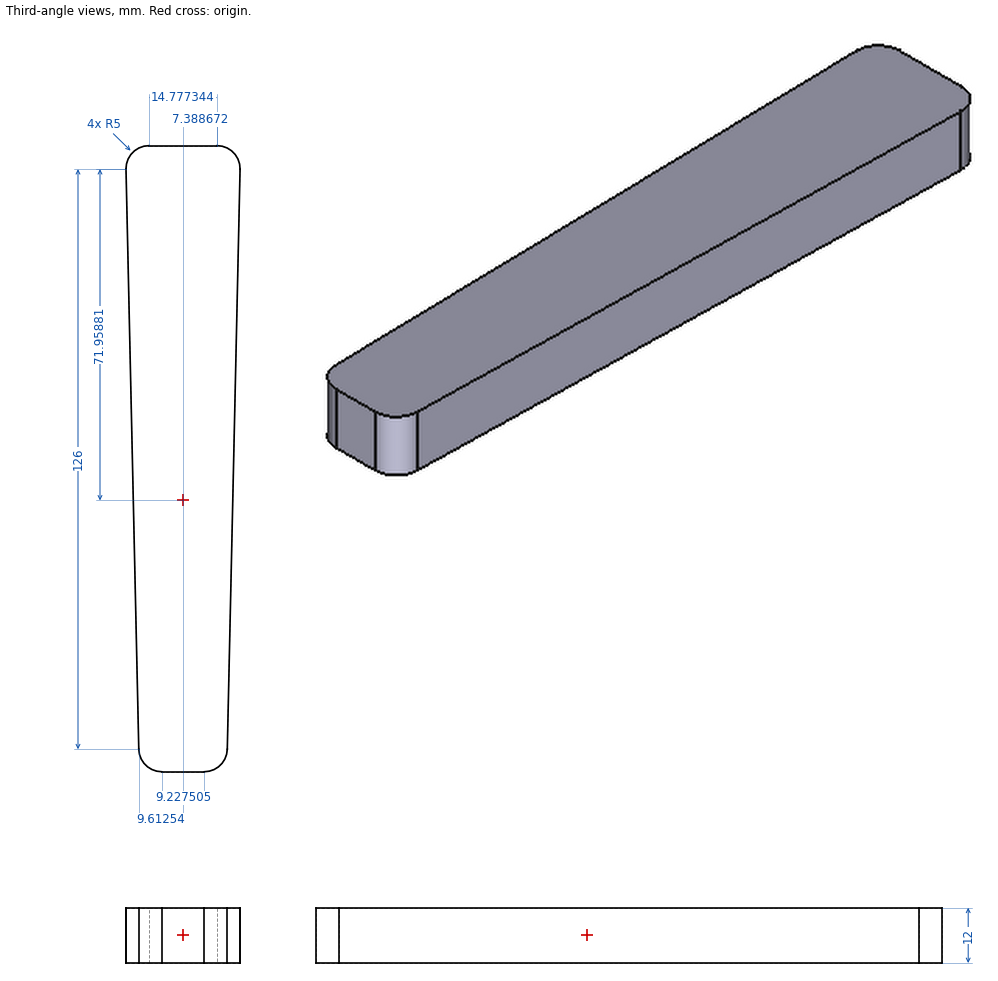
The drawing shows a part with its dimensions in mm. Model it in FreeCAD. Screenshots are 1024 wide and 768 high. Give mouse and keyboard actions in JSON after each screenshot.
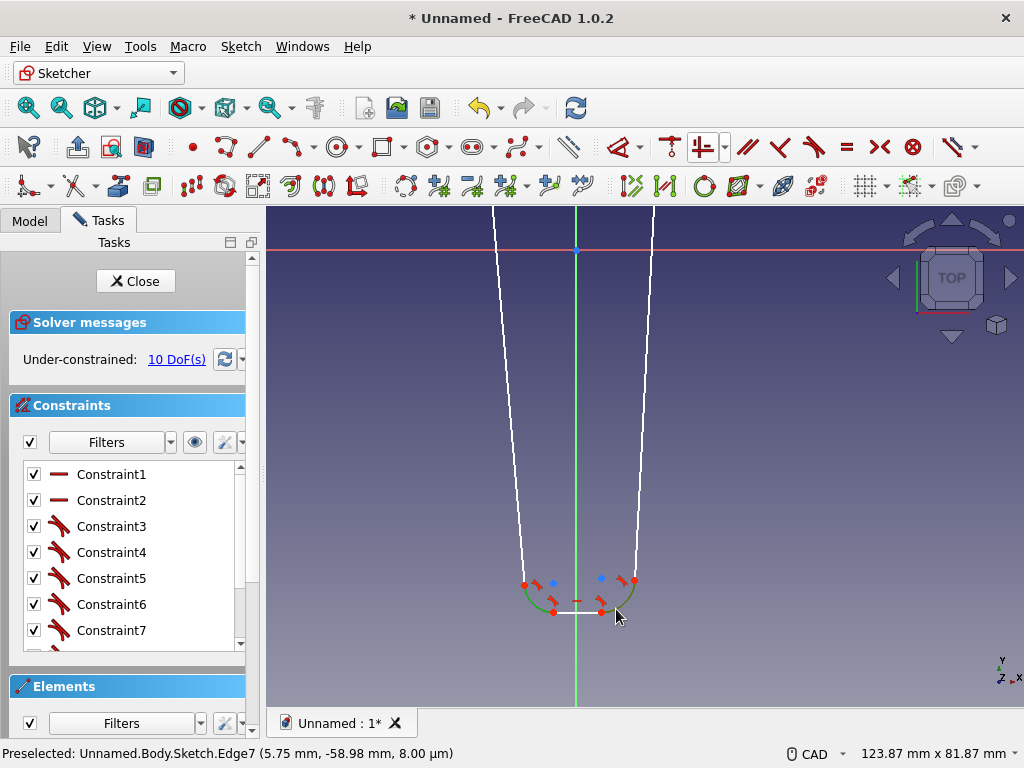
{"action": "scroll", "coordinate": [577, 609], "scroll_direction": "down", "scroll_amount": 5}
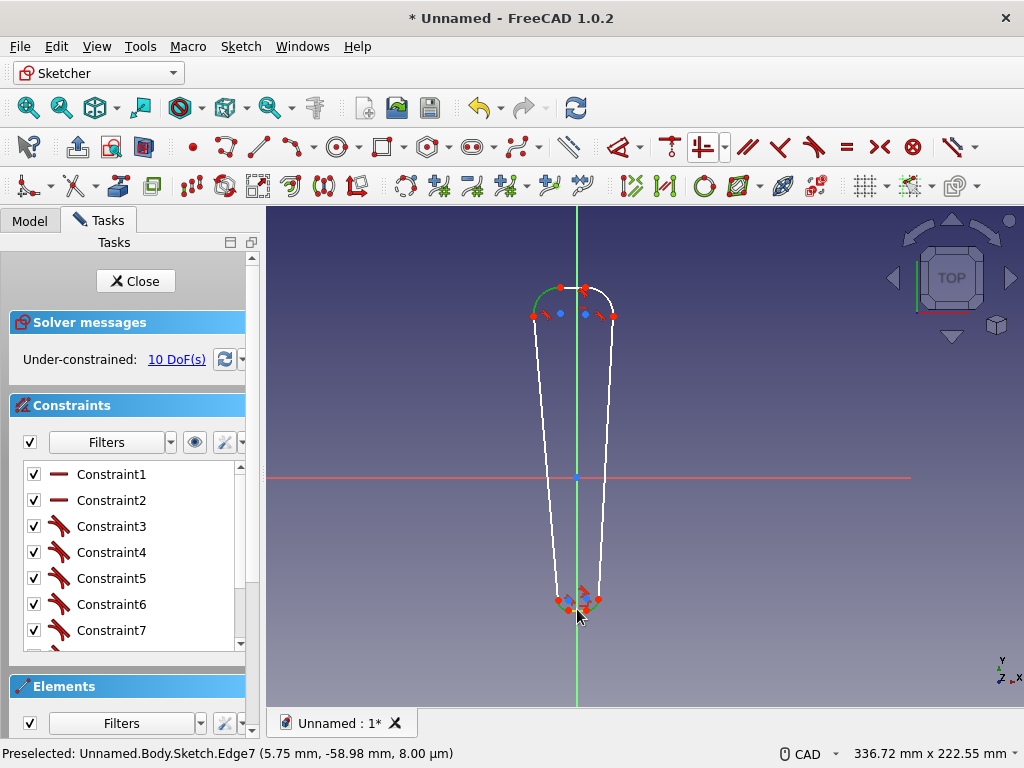
{"action": "left_click", "coordinate": [611, 303]}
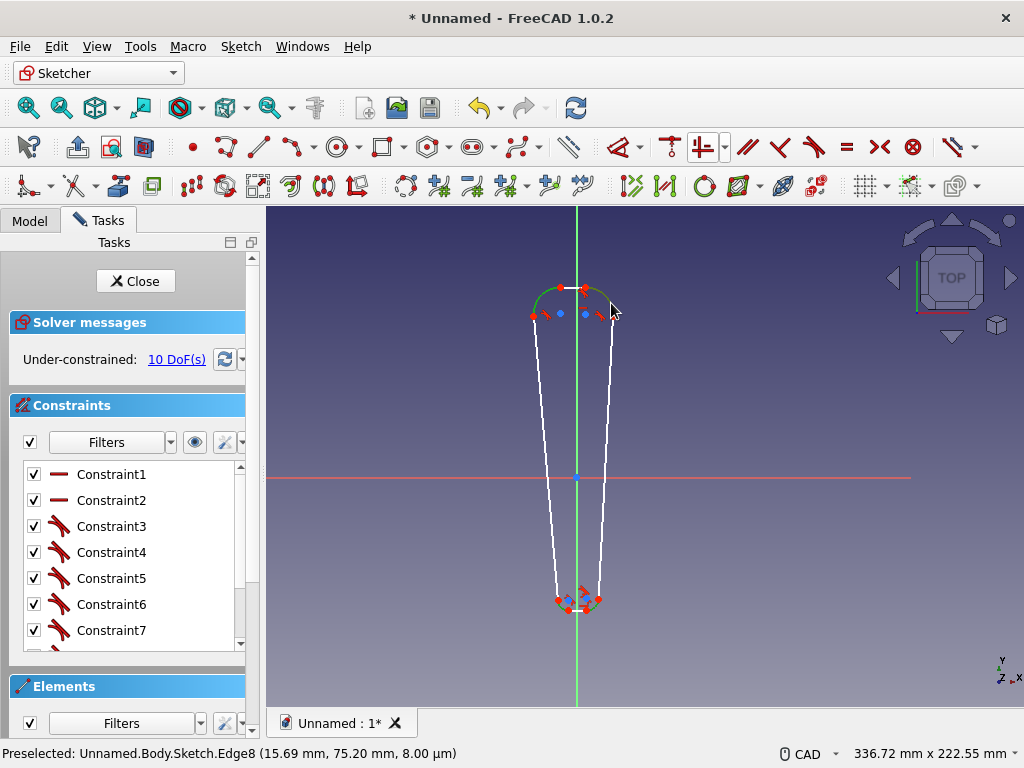
{"action": "left_click", "coordinate": [847, 148]}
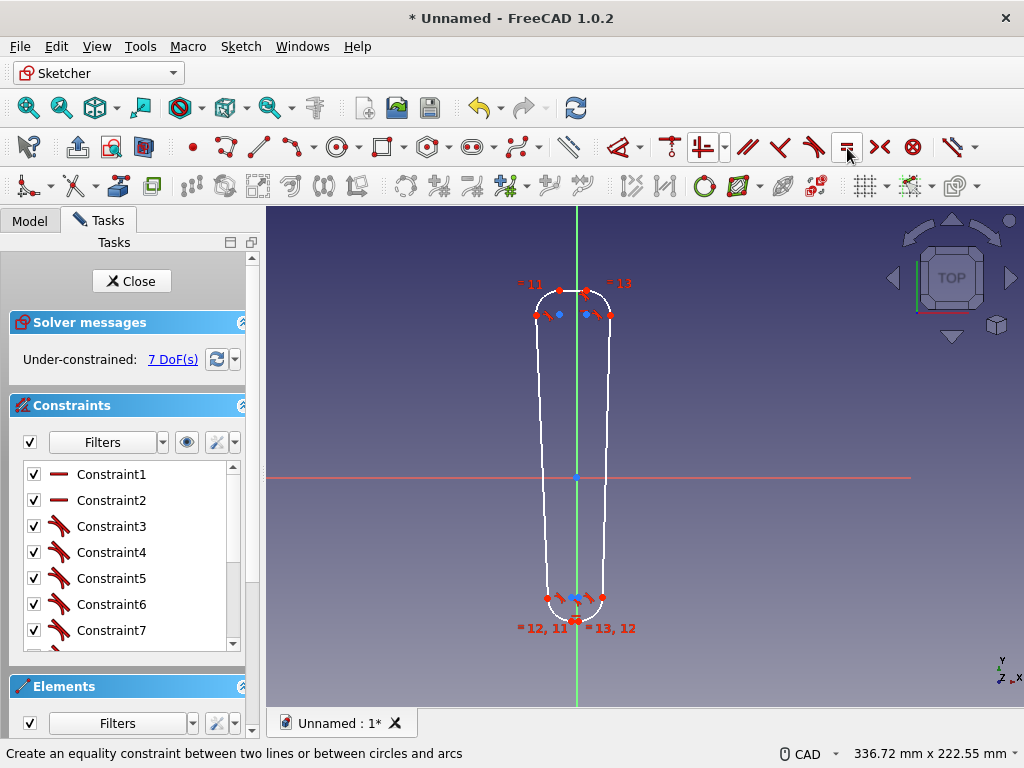
{"action": "left_click", "coordinate": [618, 148]}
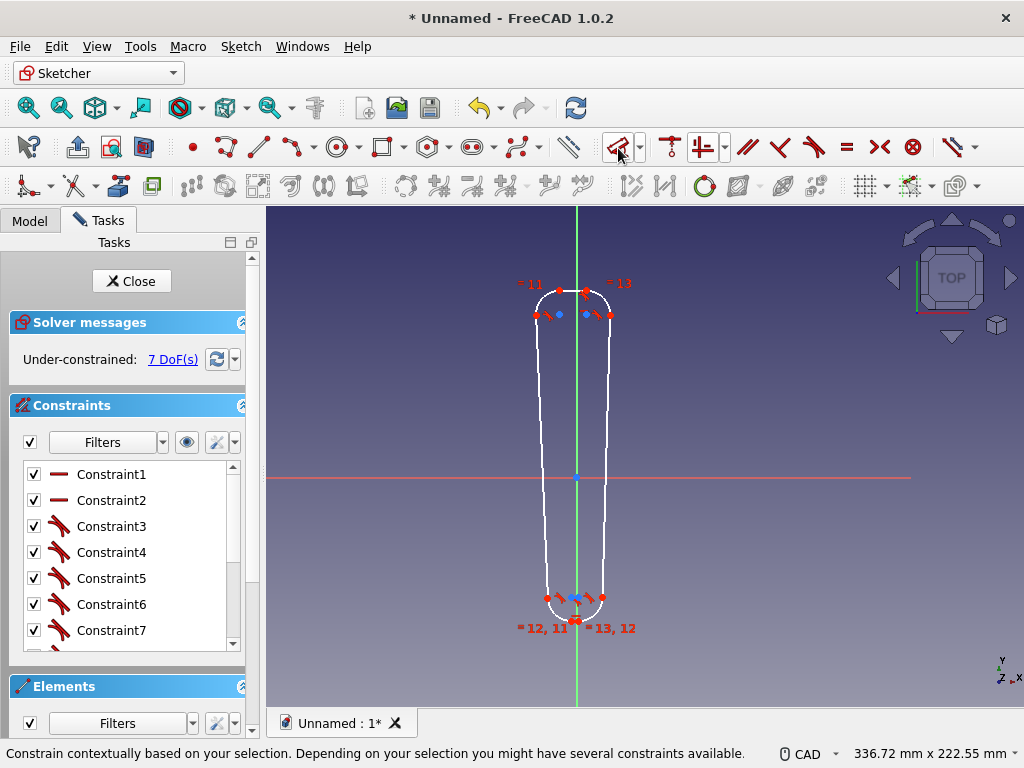
{"action": "scroll", "coordinate": [549, 293], "scroll_direction": "up", "scroll_amount": 7}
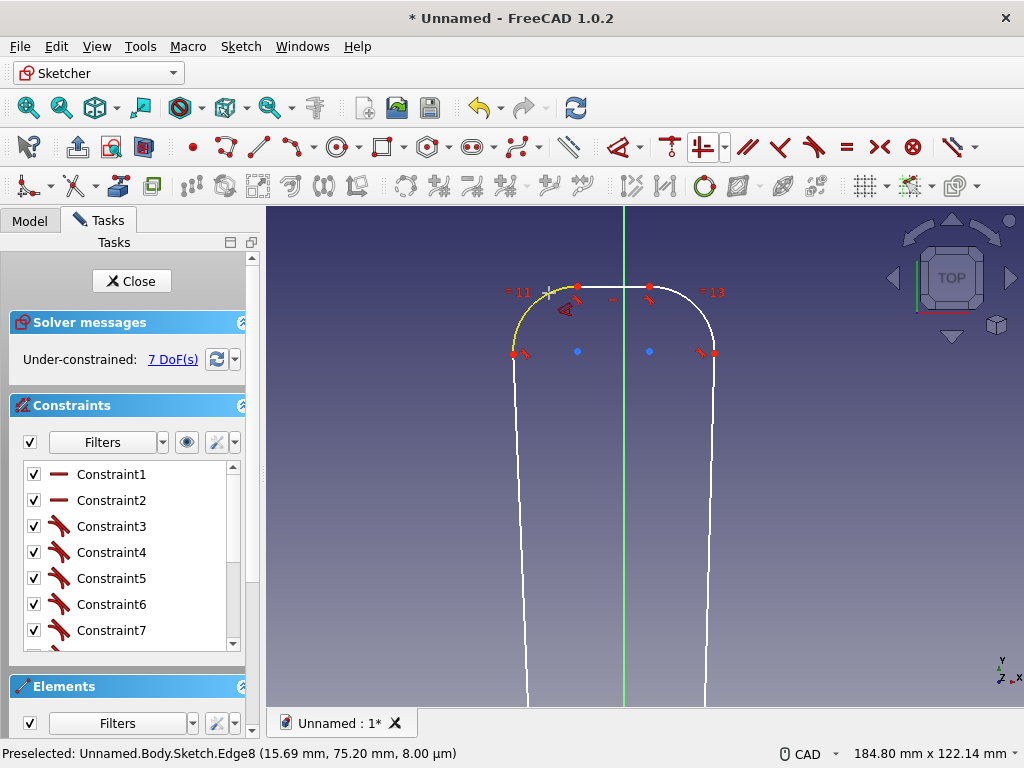
{"action": "left_click", "coordinate": [547, 294]}
{"action": "left_click", "coordinate": [532, 266]}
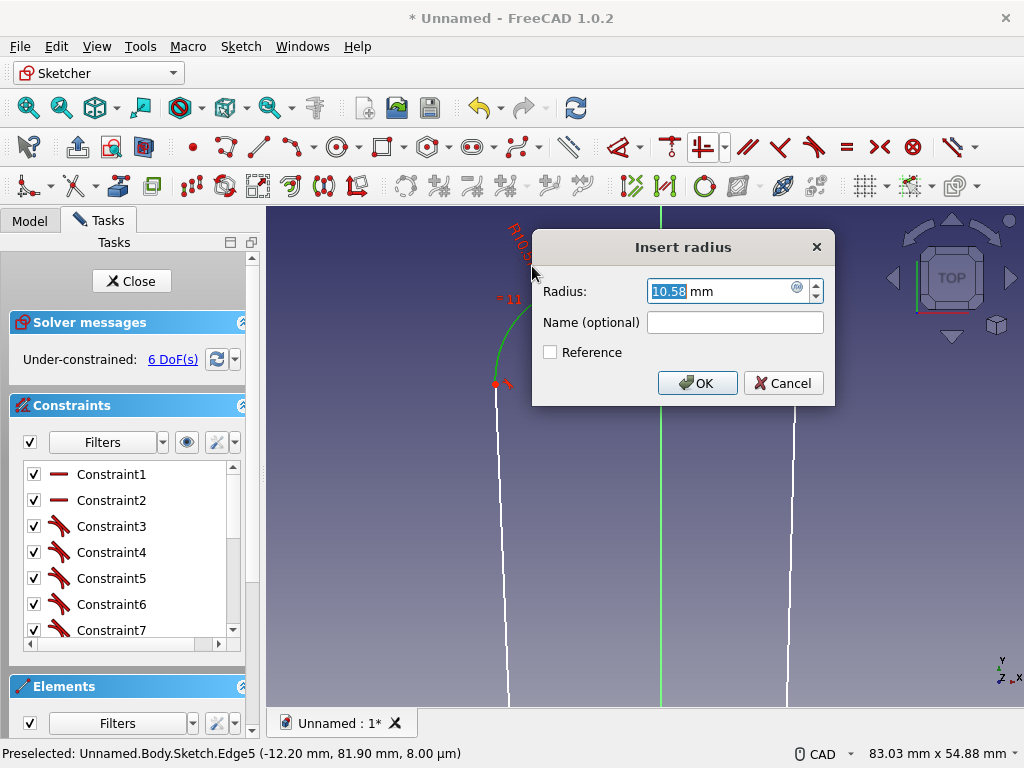
{"action": "type", "text": "5"}
{"action": "key", "text": "Return"}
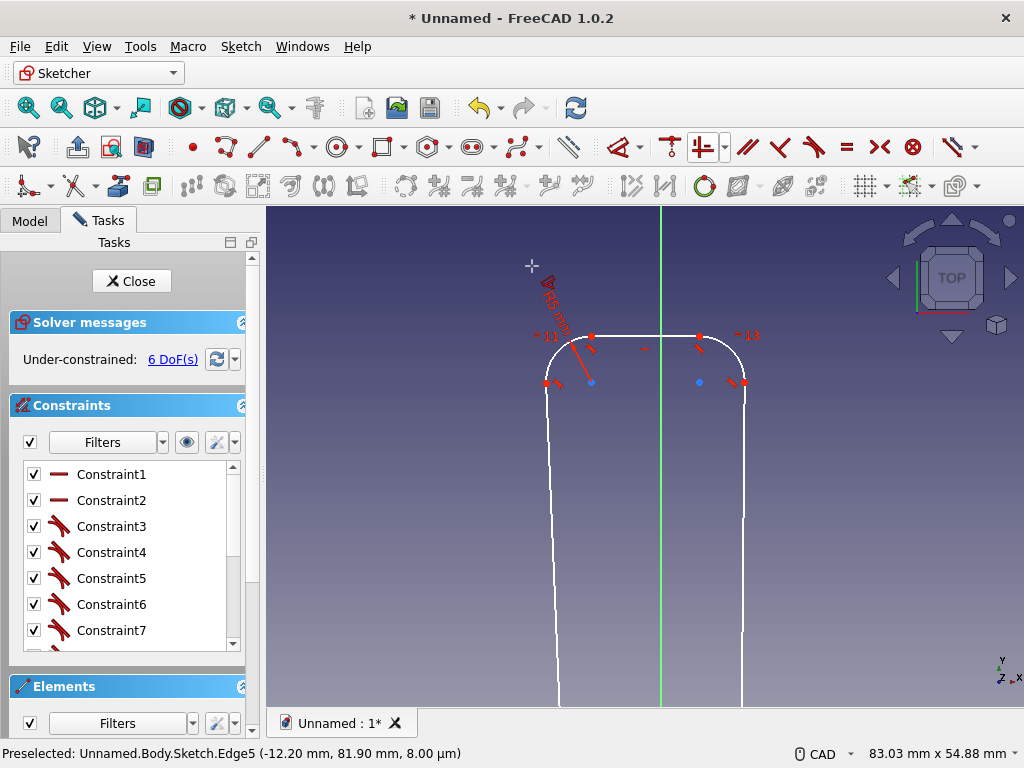
{"action": "scroll", "coordinate": [549, 292], "scroll_direction": "down", "scroll_amount": 7}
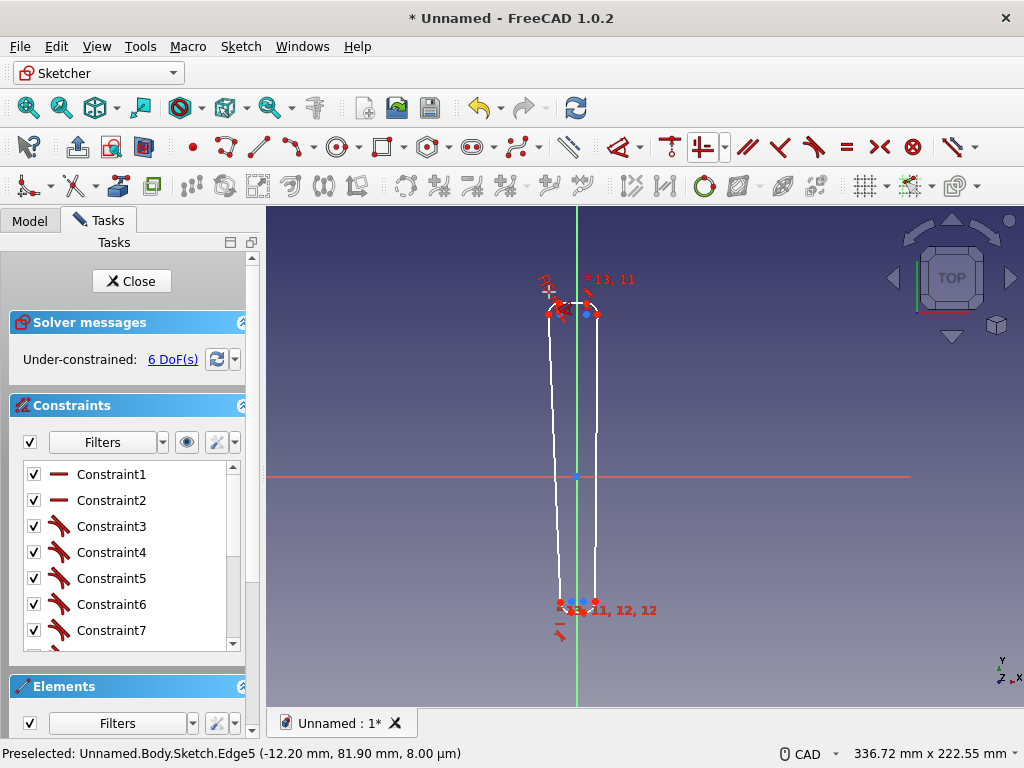
{"action": "left_click", "coordinate": [551, 372]}
{"action": "left_click", "coordinate": [515, 459]}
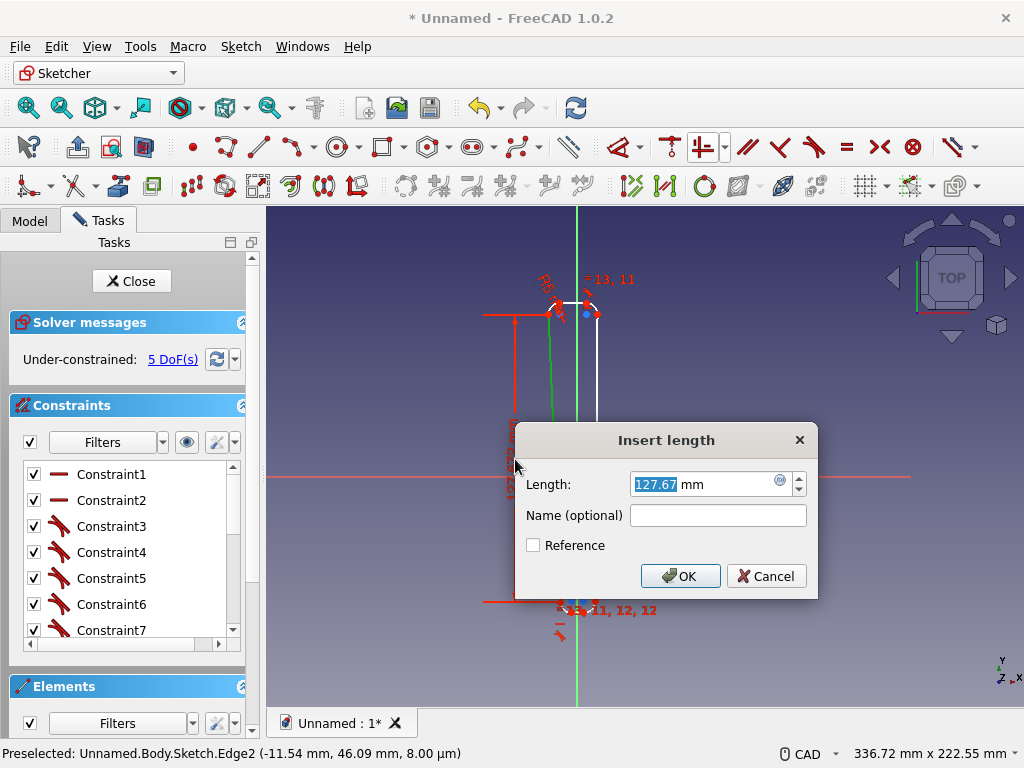
{"action": "type", "text": "126"}
{"action": "key", "text": "Return"}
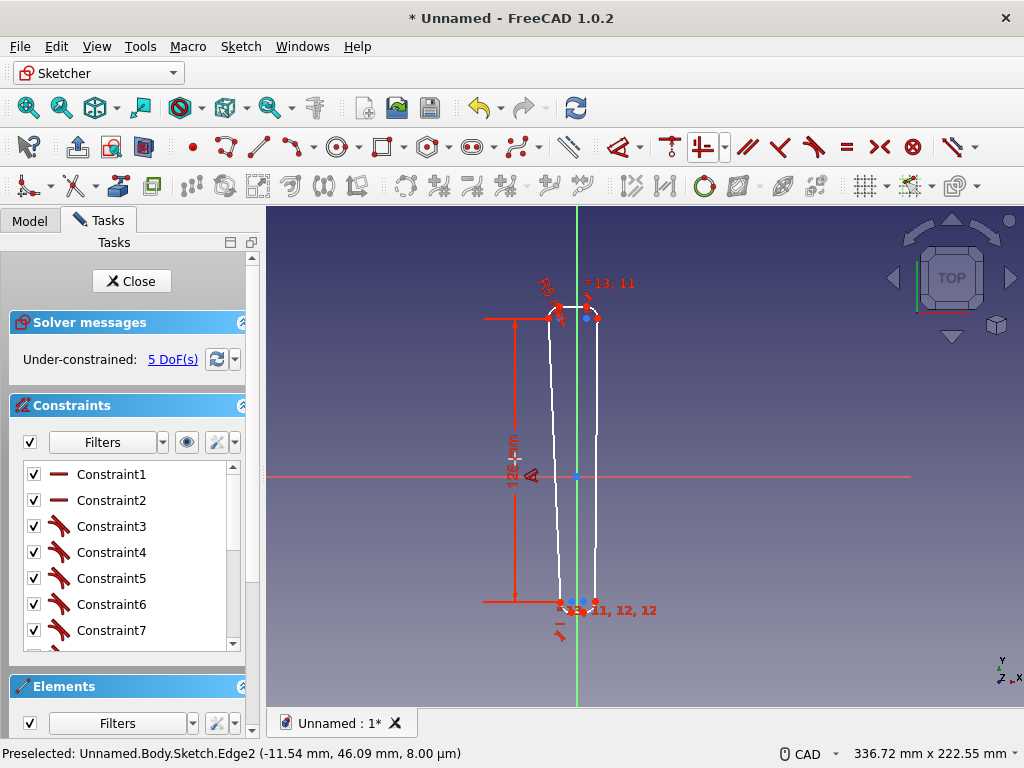
{"action": "scroll", "coordinate": [578, 613], "scroll_direction": "up", "scroll_amount": 5}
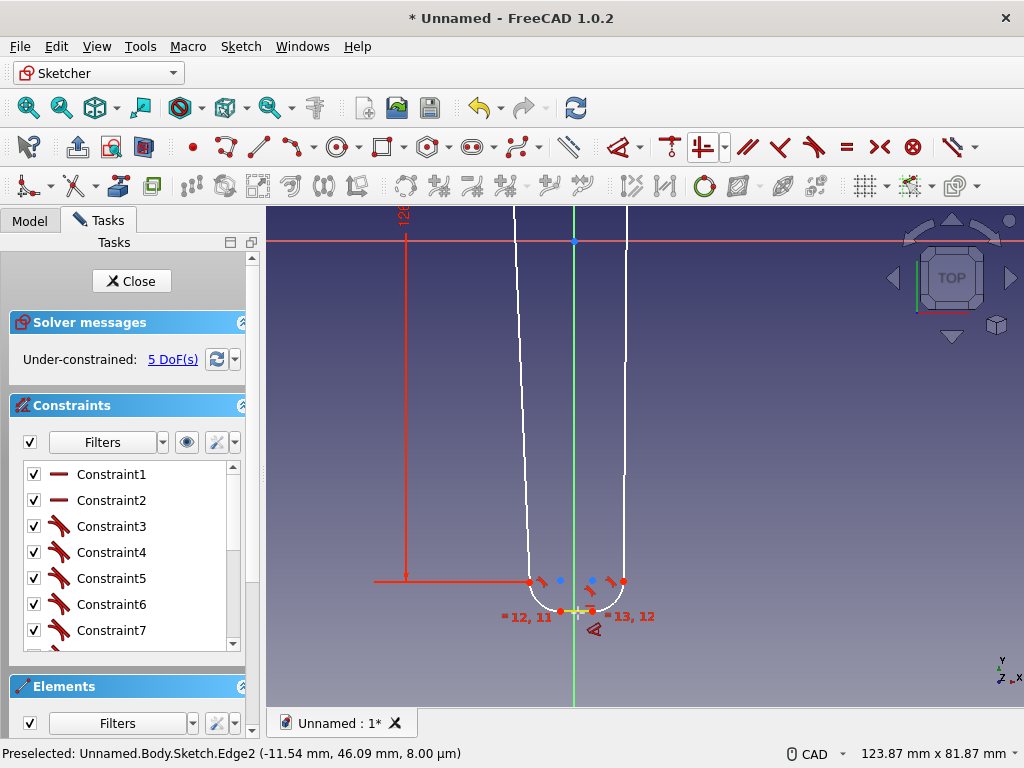
{"action": "left_click", "coordinate": [577, 611]}
{"action": "left_click", "coordinate": [588, 645]}